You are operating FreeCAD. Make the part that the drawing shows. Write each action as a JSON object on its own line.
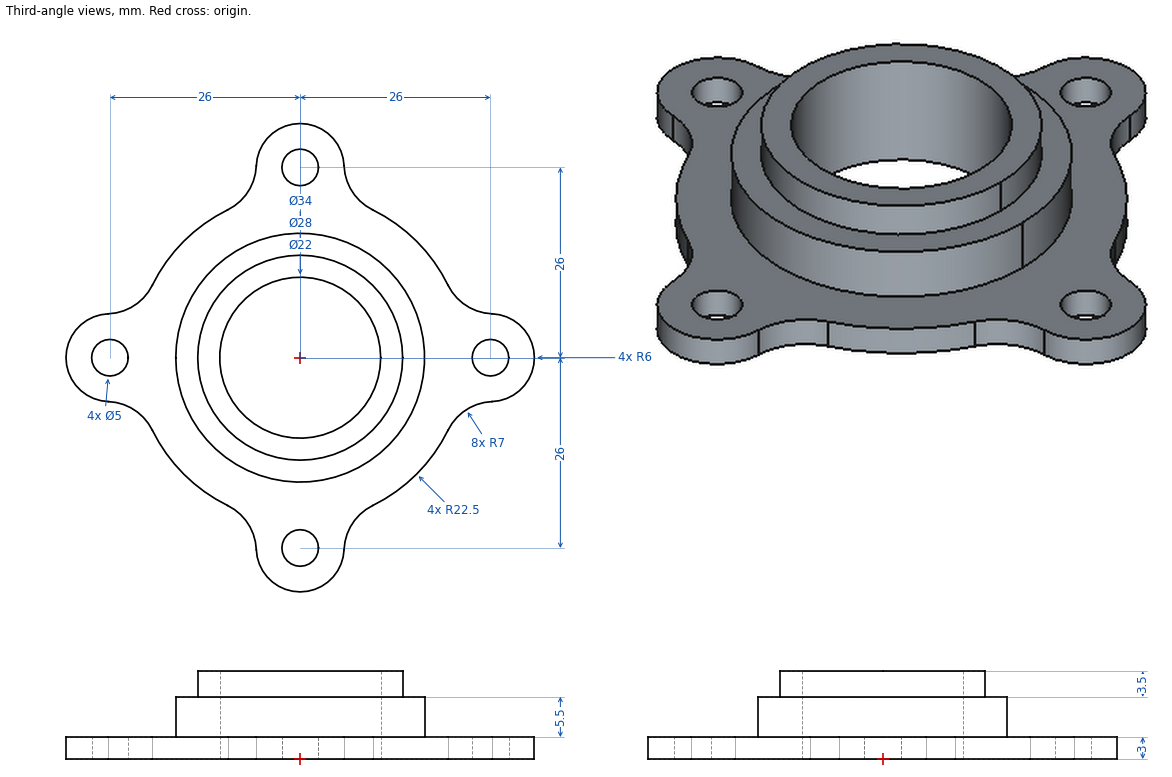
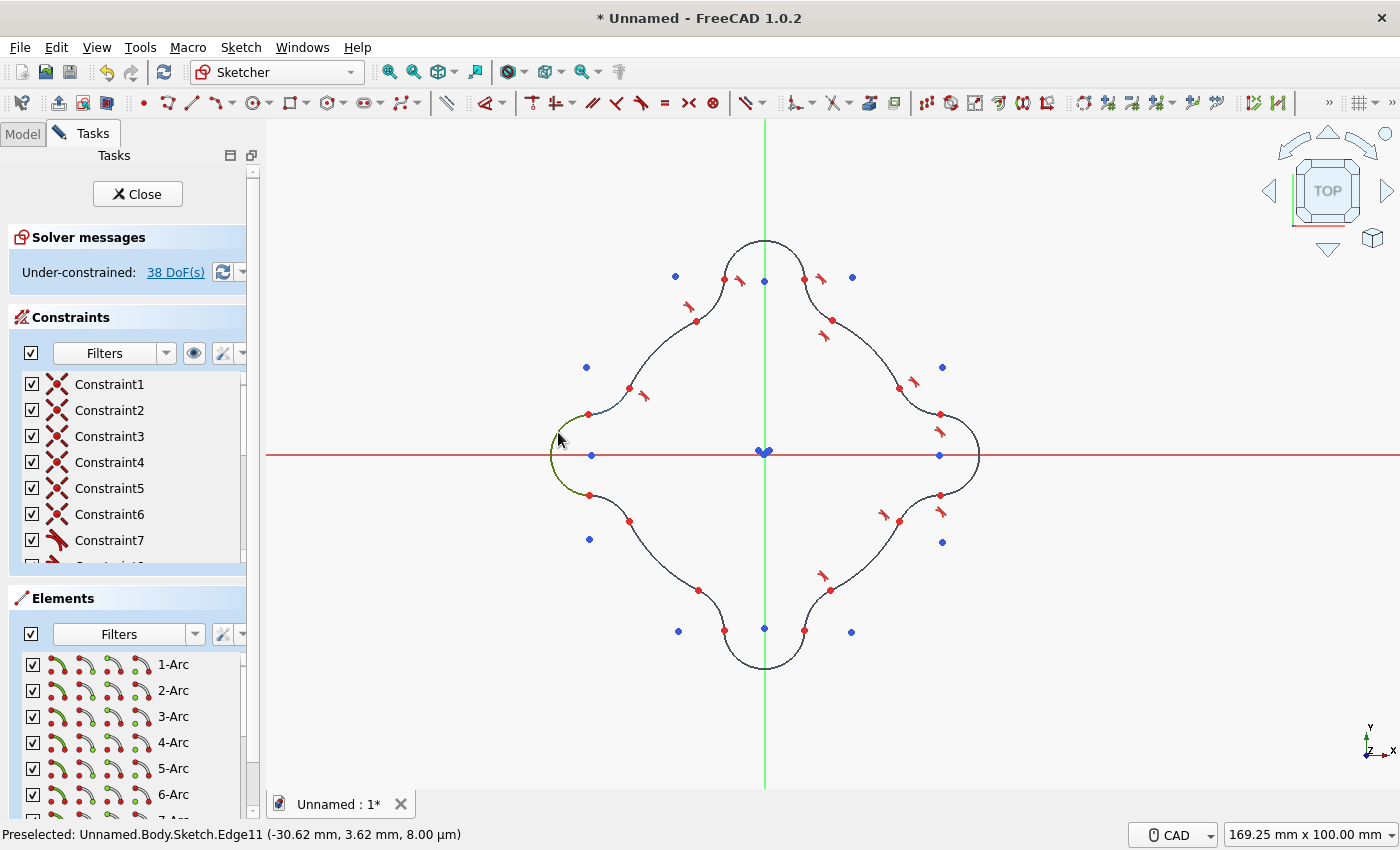
{"action": "left_click", "coordinate": [642, 104]}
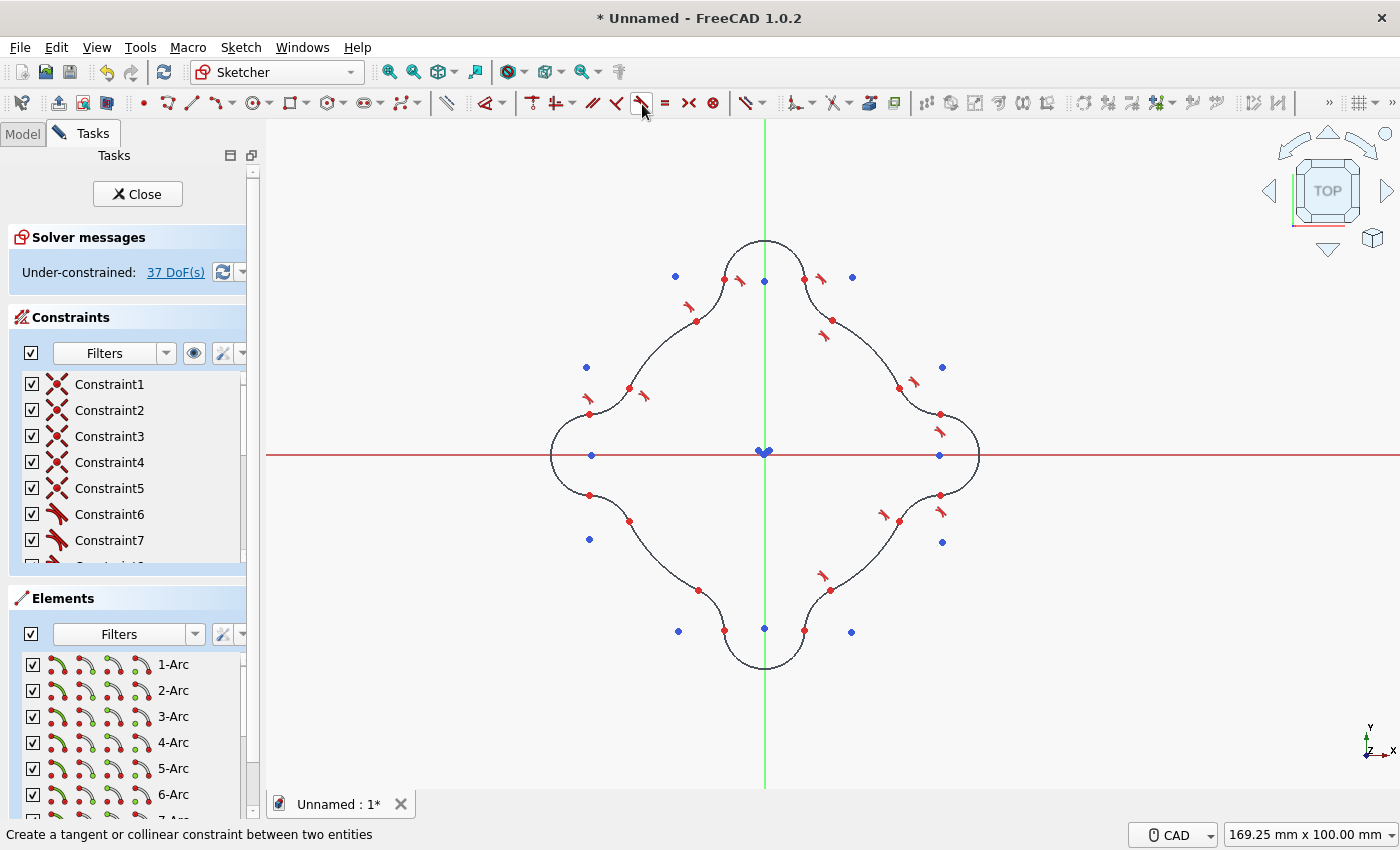
{"action": "left_click", "coordinate": [558, 432]}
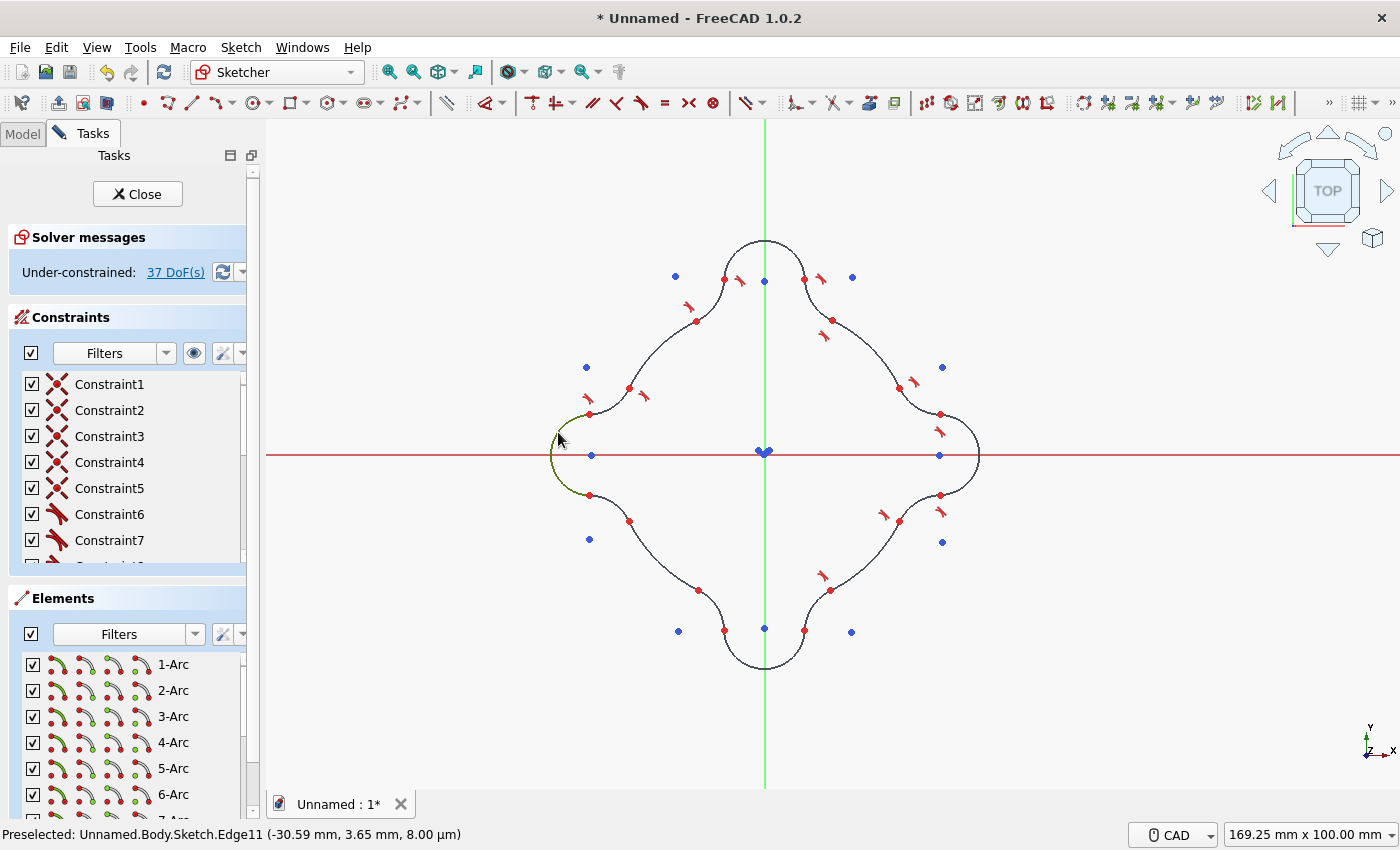
{"action": "left_click", "coordinate": [621, 509]}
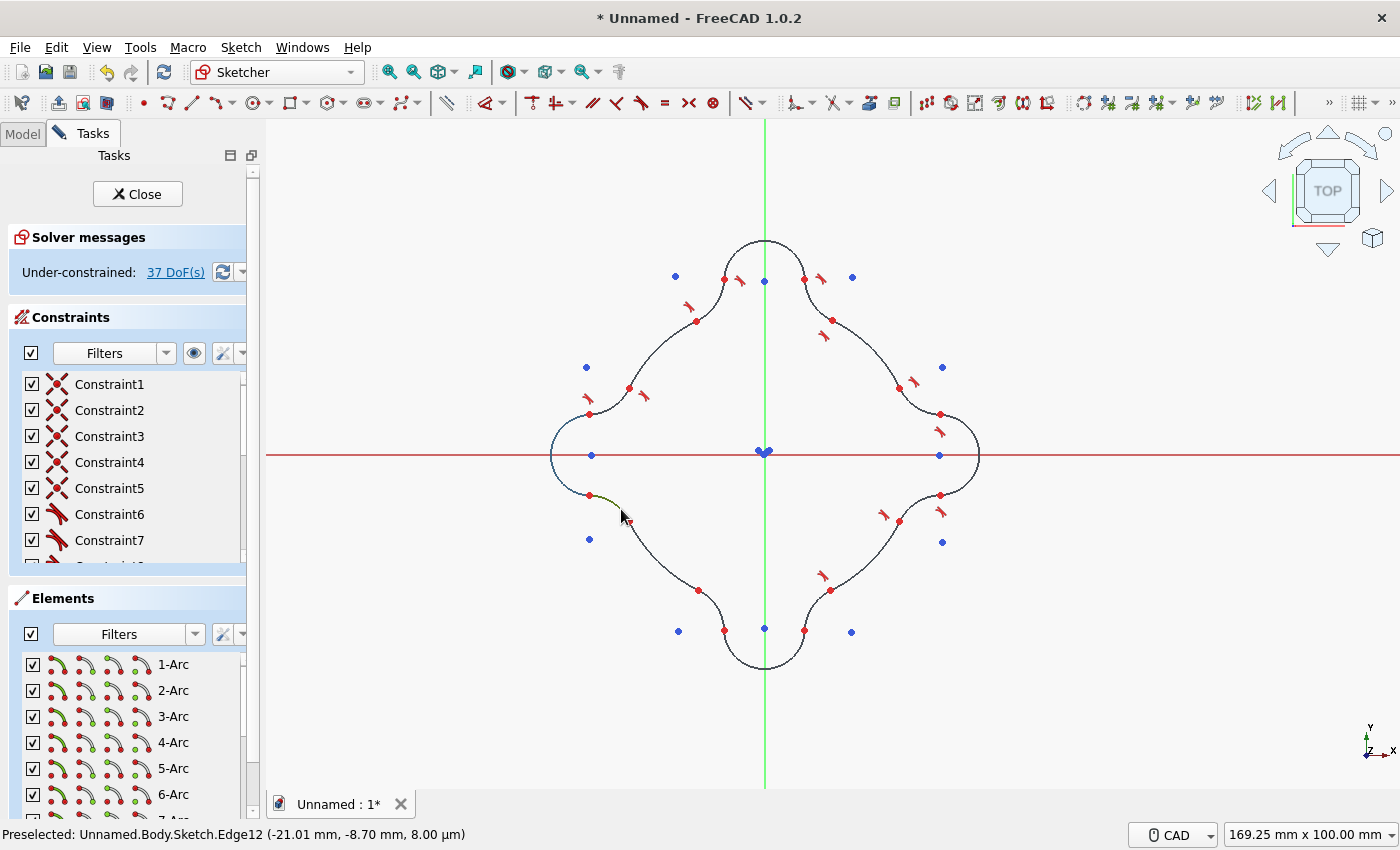
{"action": "left_click", "coordinate": [642, 104]}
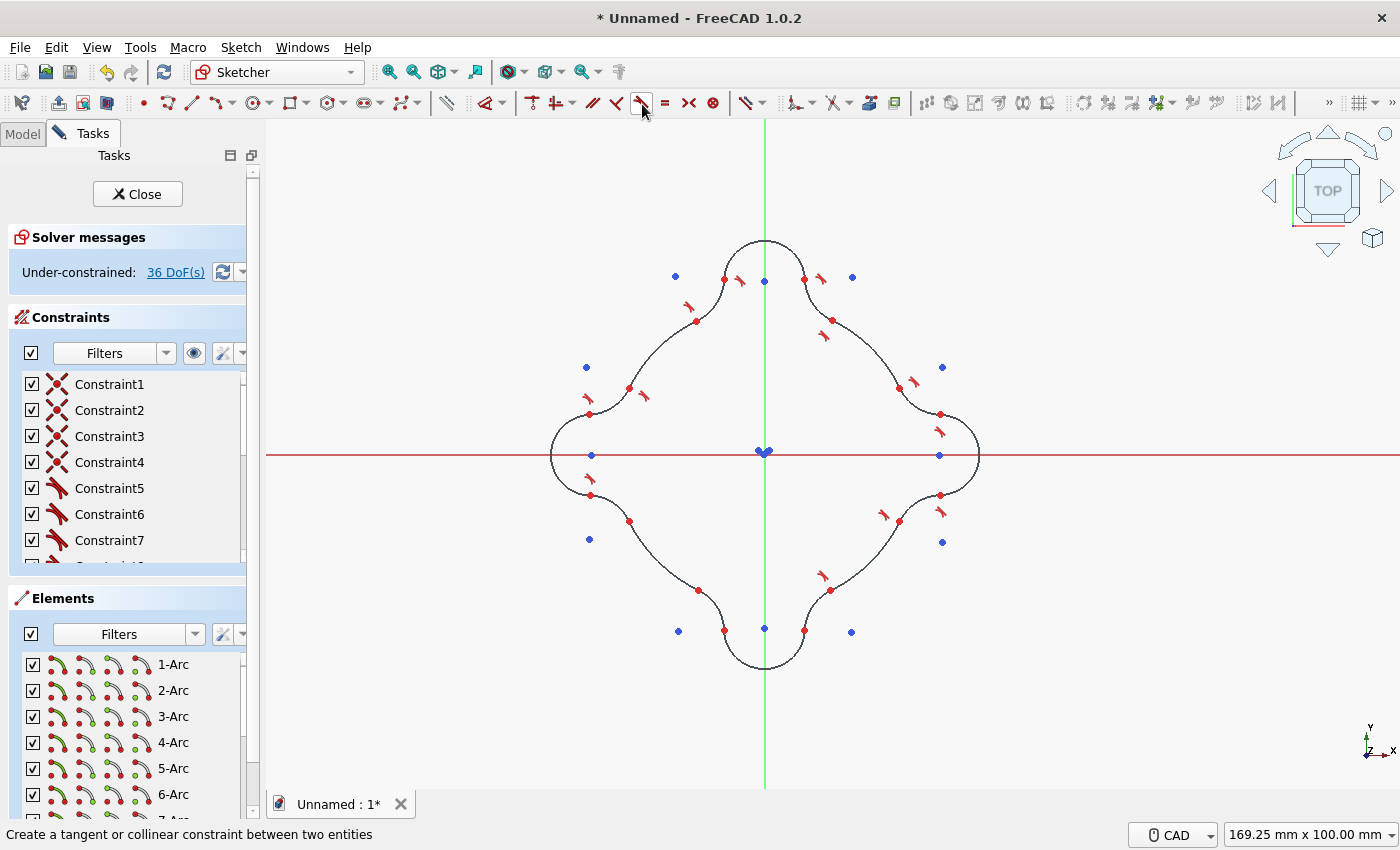
{"action": "left_click", "coordinate": [621, 509]}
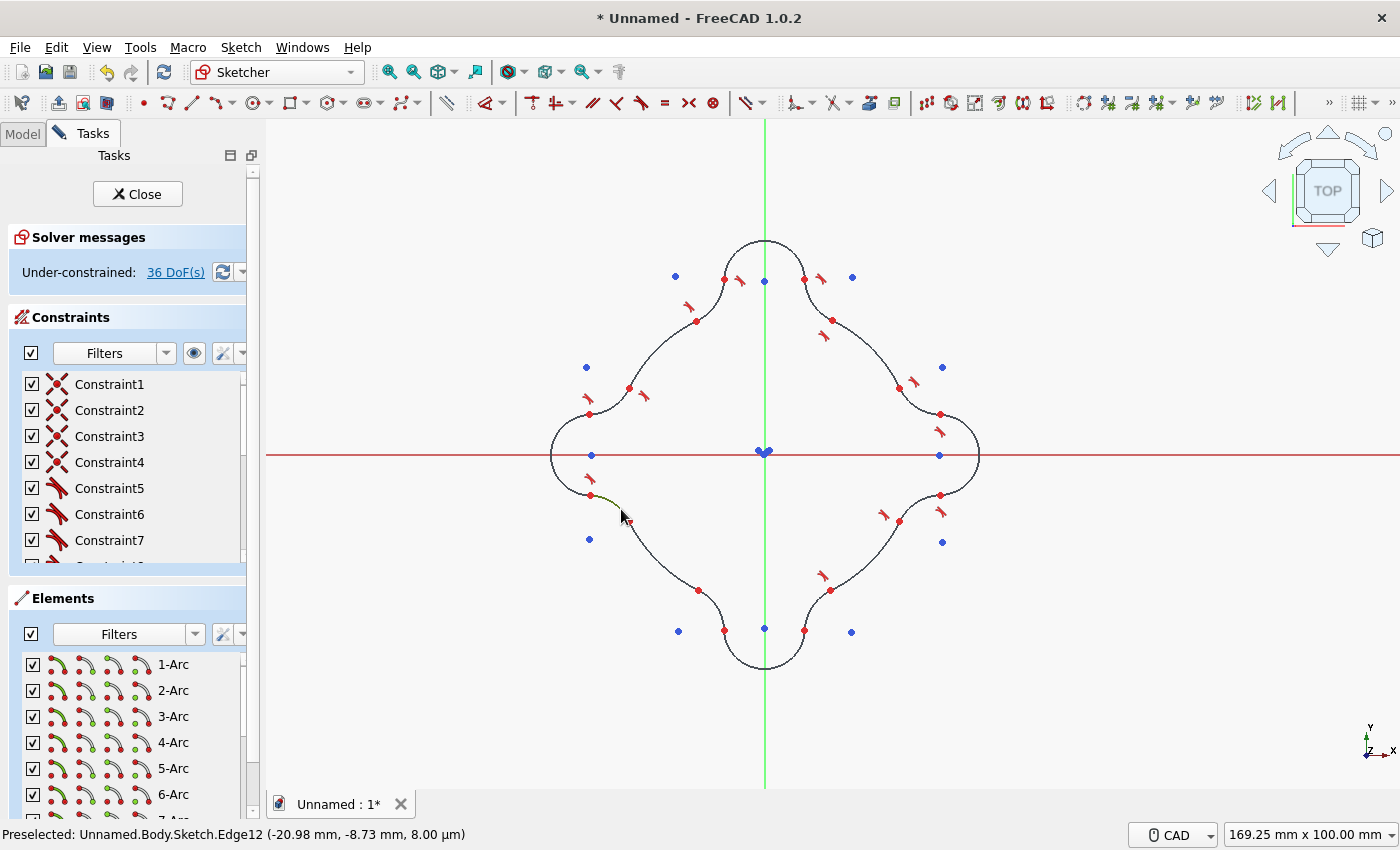
{"action": "left_click", "coordinate": [645, 547]}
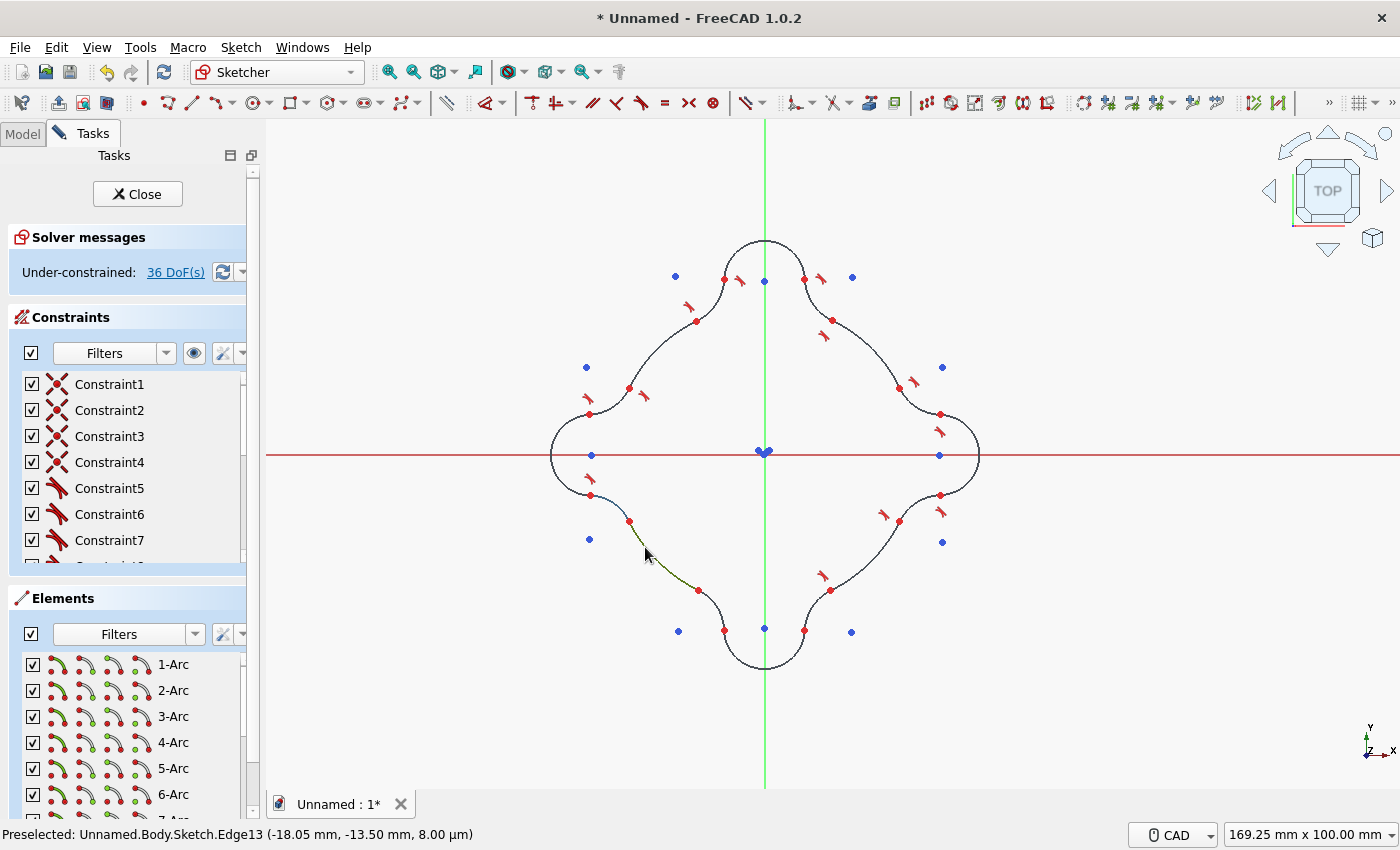
{"action": "left_click", "coordinate": [642, 104]}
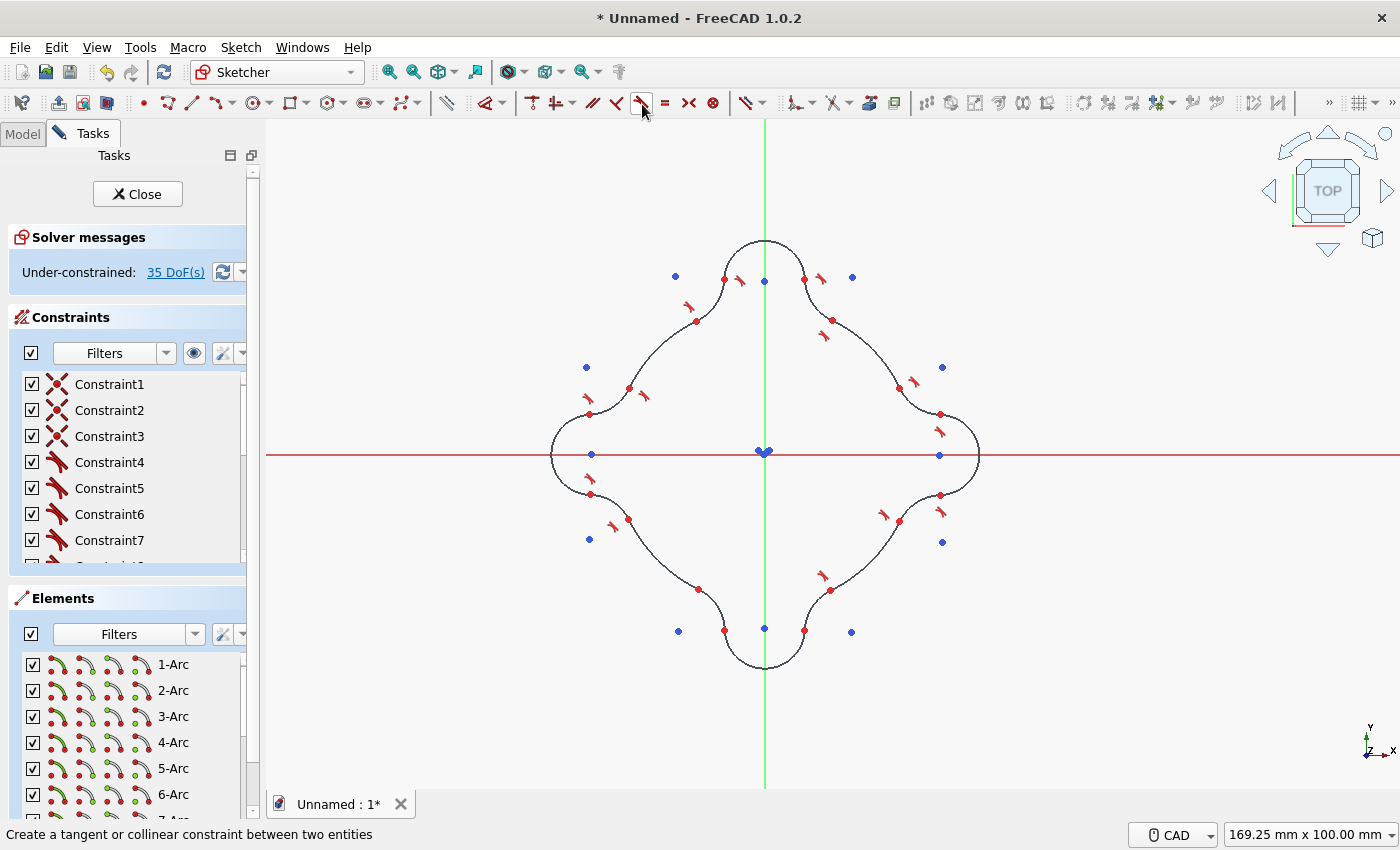
{"action": "left_click", "coordinate": [645, 545]}